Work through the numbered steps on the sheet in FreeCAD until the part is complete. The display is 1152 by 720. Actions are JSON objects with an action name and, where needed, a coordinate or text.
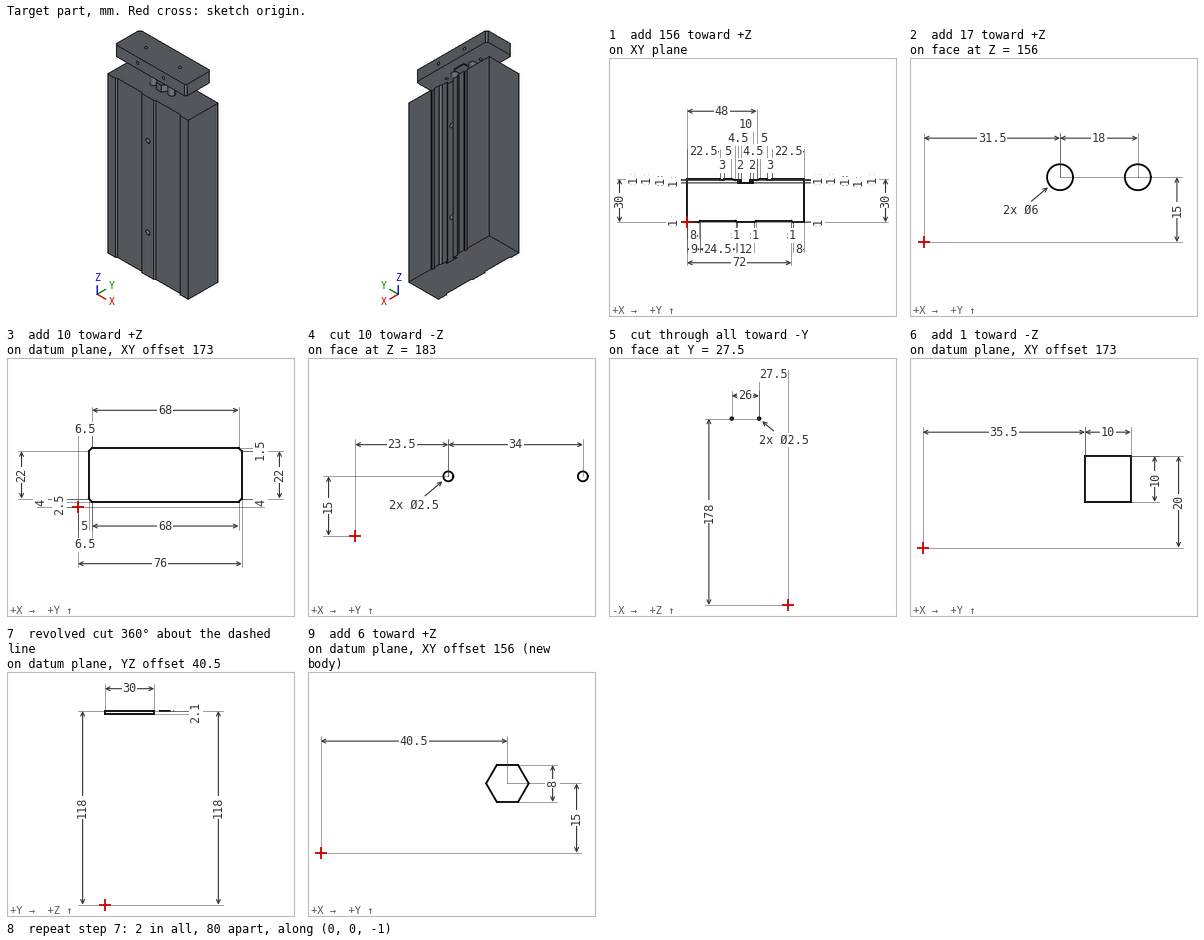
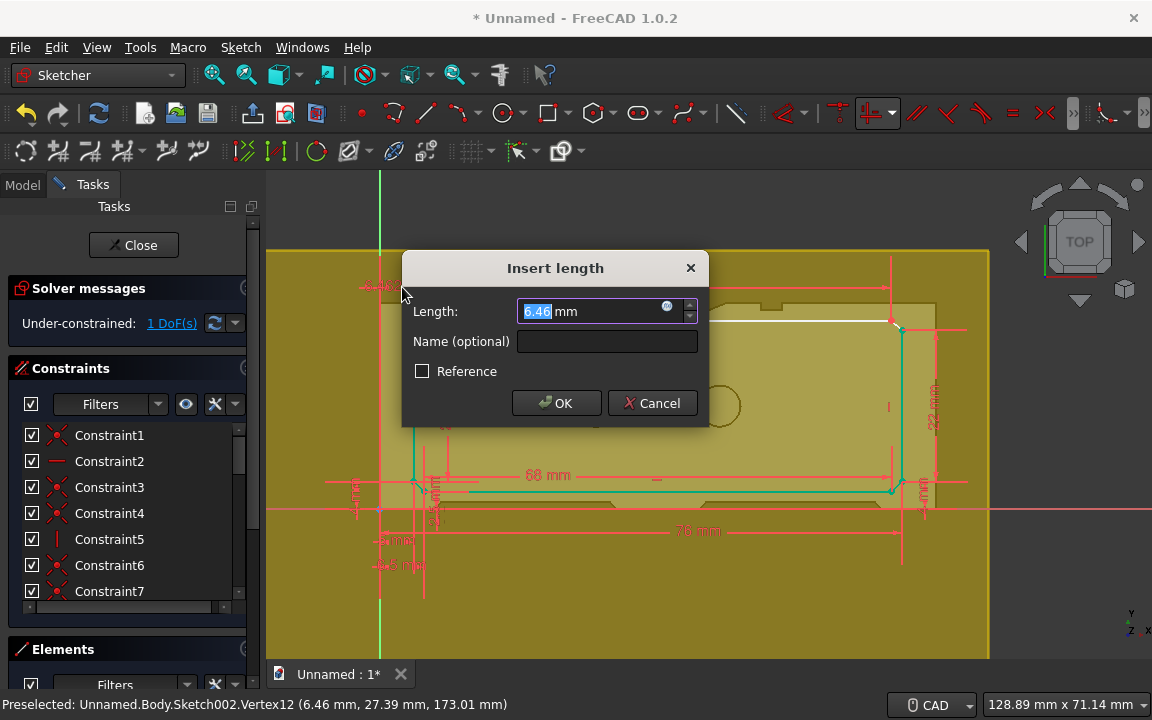
{"action": "type", "text": "6.5"}
{"action": "key", "text": "Return"}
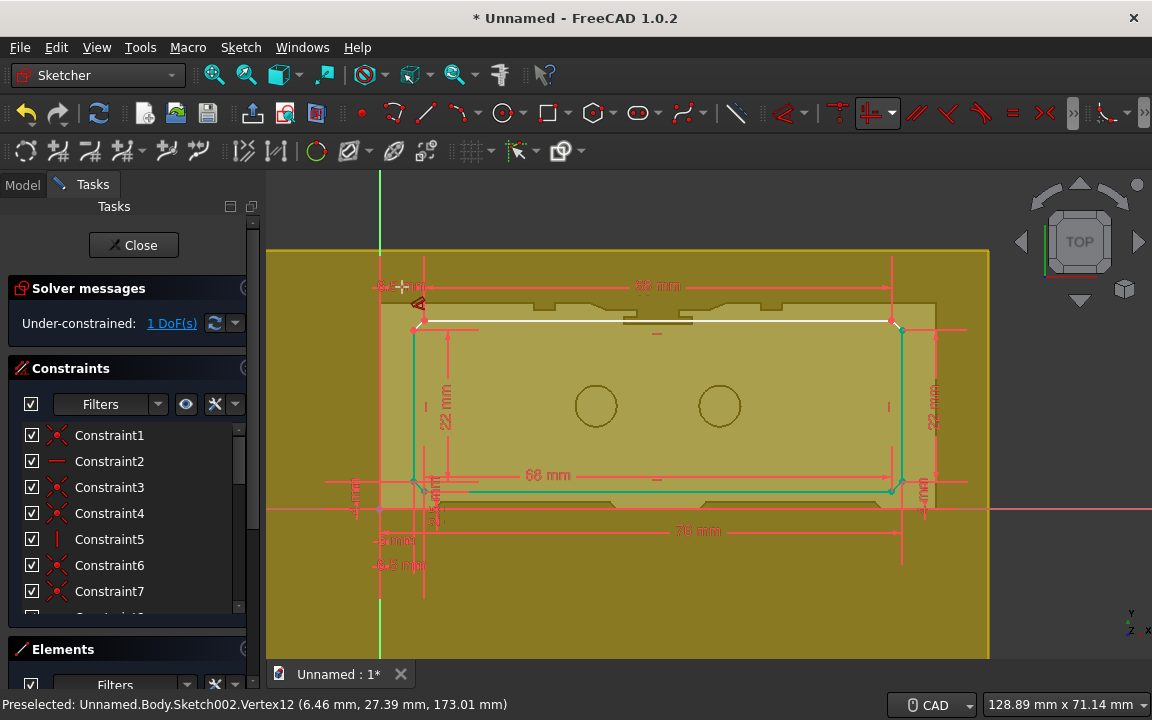
{"action": "scroll", "coordinate": [897, 326], "scroll_direction": "up", "scroll_amount": 7}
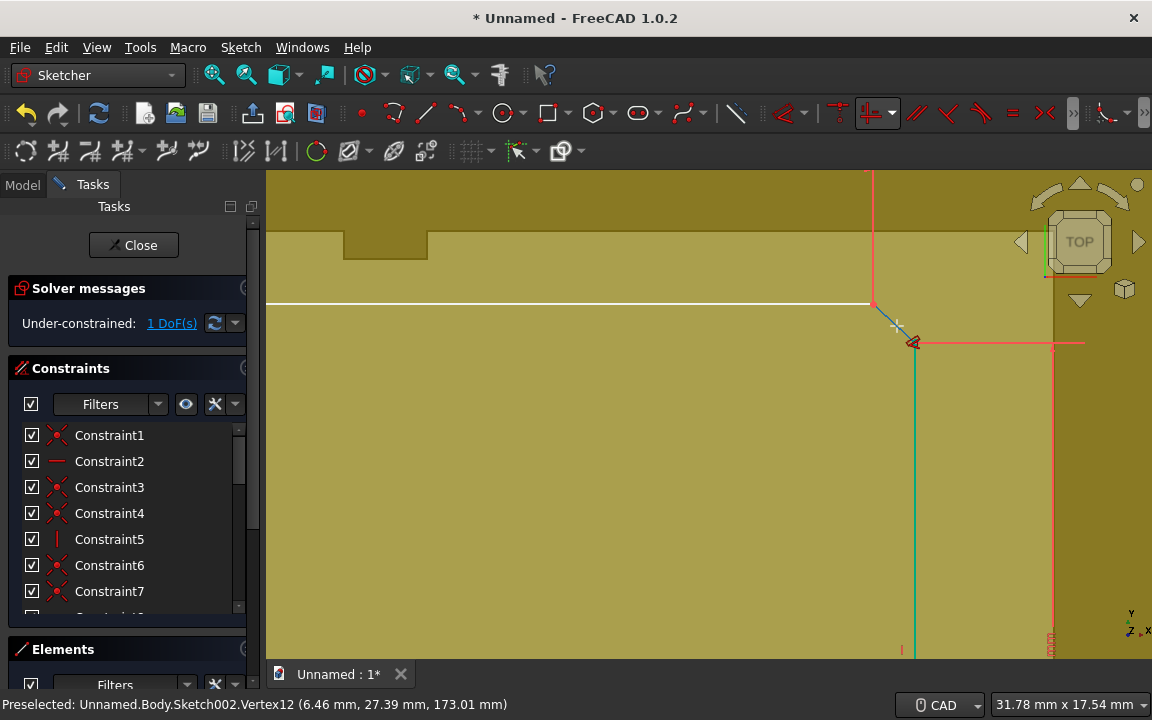
{"action": "left_click", "coordinate": [894, 324]}
{"action": "left_click", "coordinate": [949, 324]}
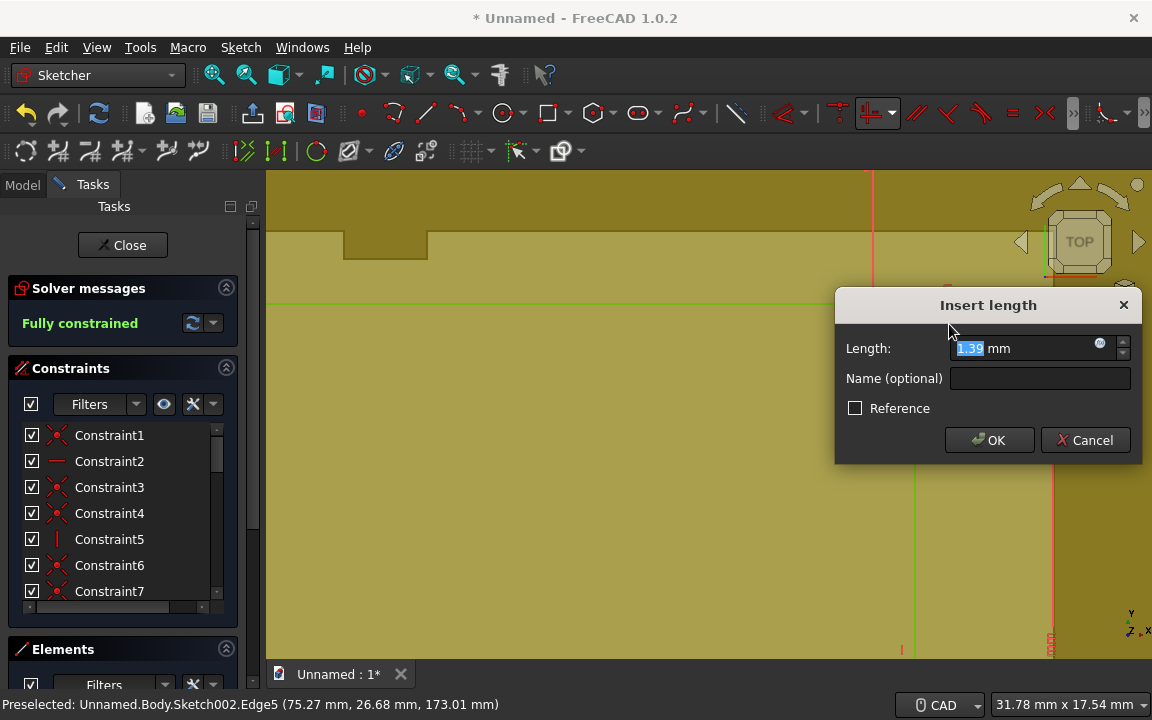
{"action": "type", "text": "1.5"}
{"action": "key", "text": "Return"}
{"action": "key", "text": "Escape"}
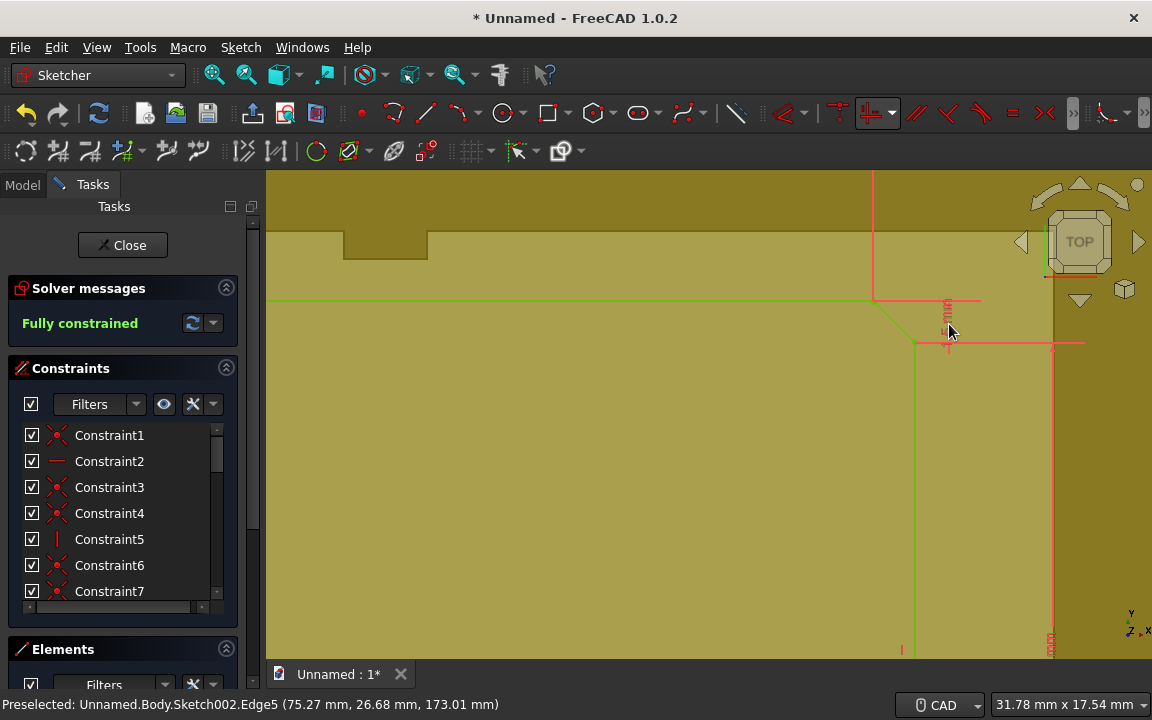
{"action": "left_click", "coordinate": [123, 245]}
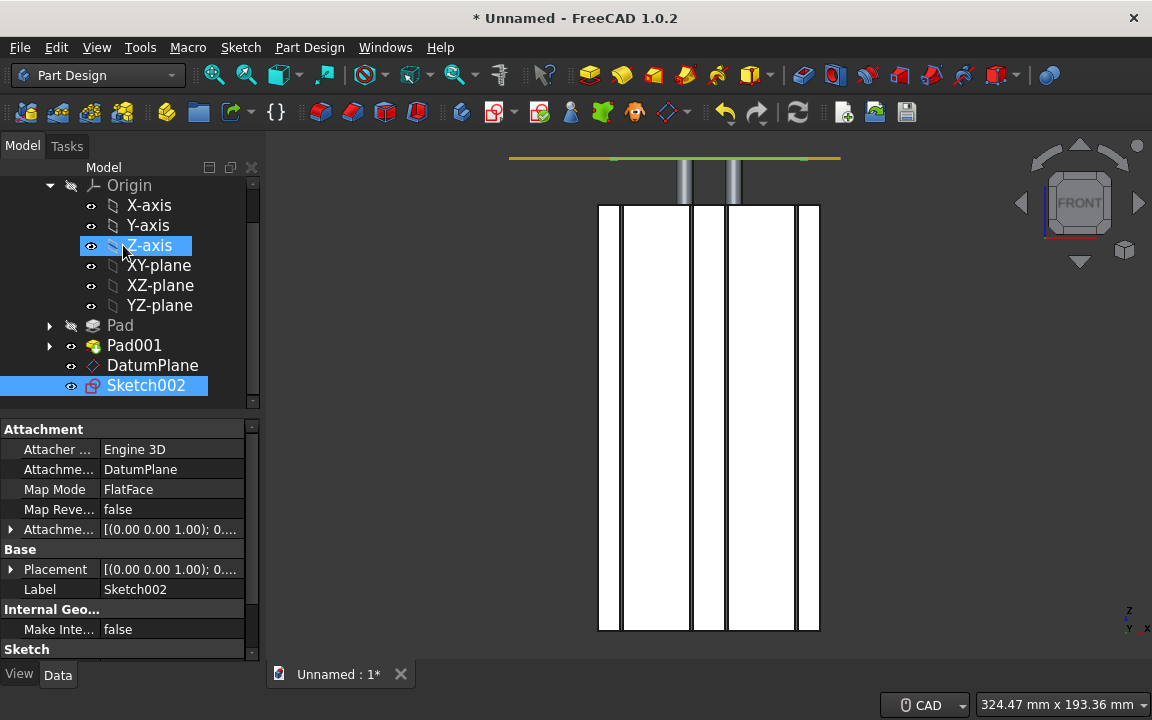
{"action": "left_click", "coordinate": [590, 76]}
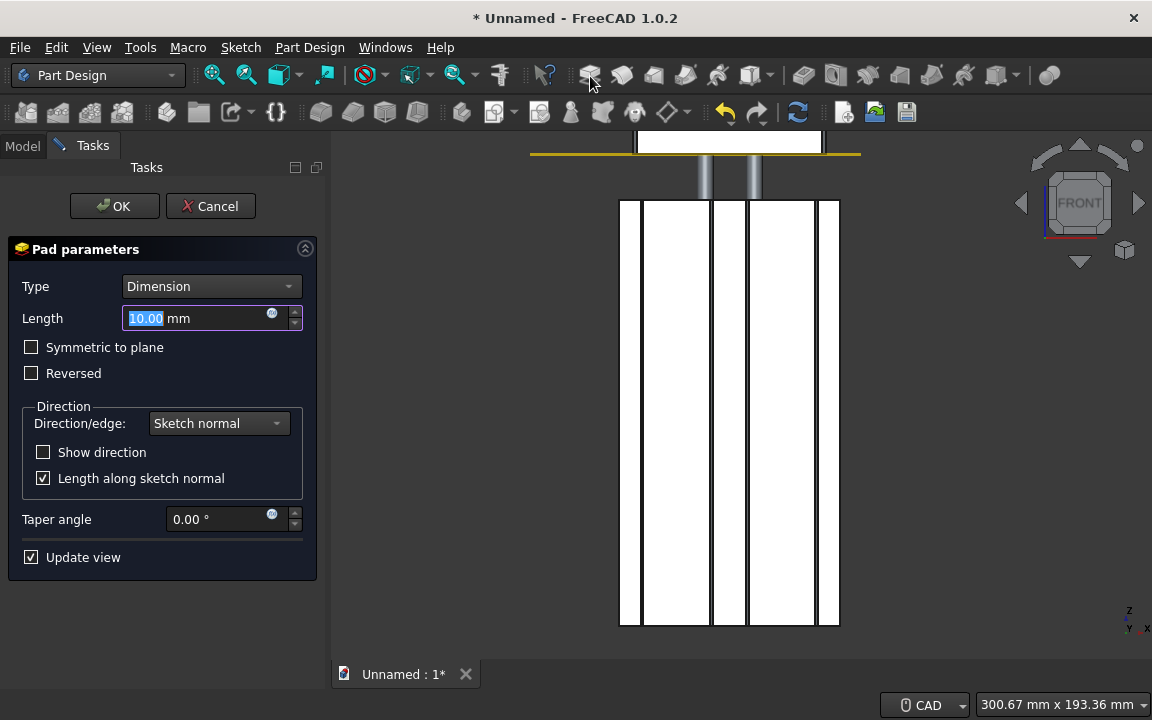
{"action": "type", "text": "10"}
{"action": "key", "text": "Tab"}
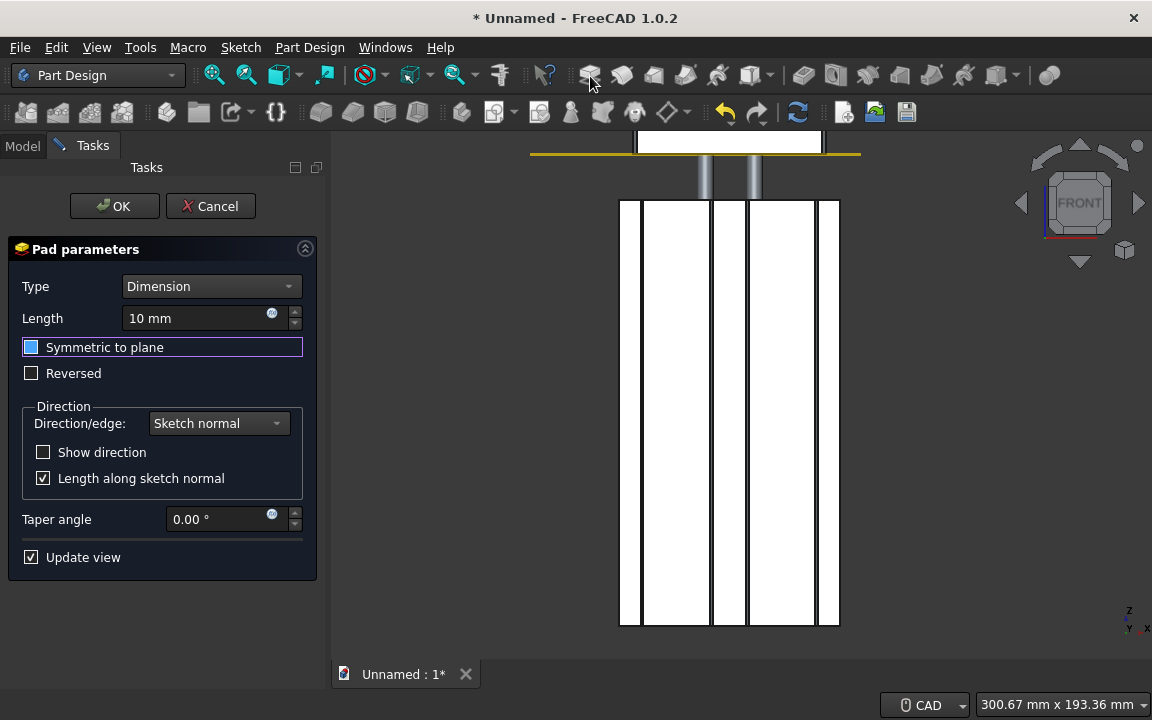
{"action": "left_click", "coordinate": [115, 206]}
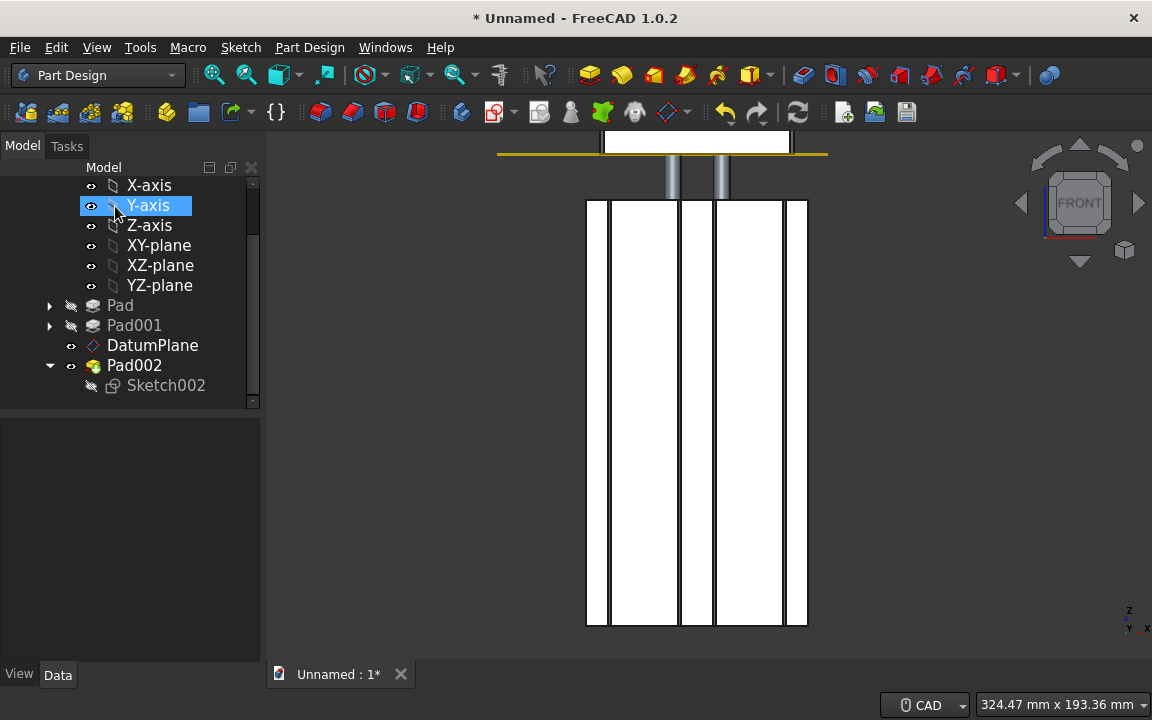
{"action": "left_click", "coordinate": [116, 346]}
{"action": "key", "text": "space"}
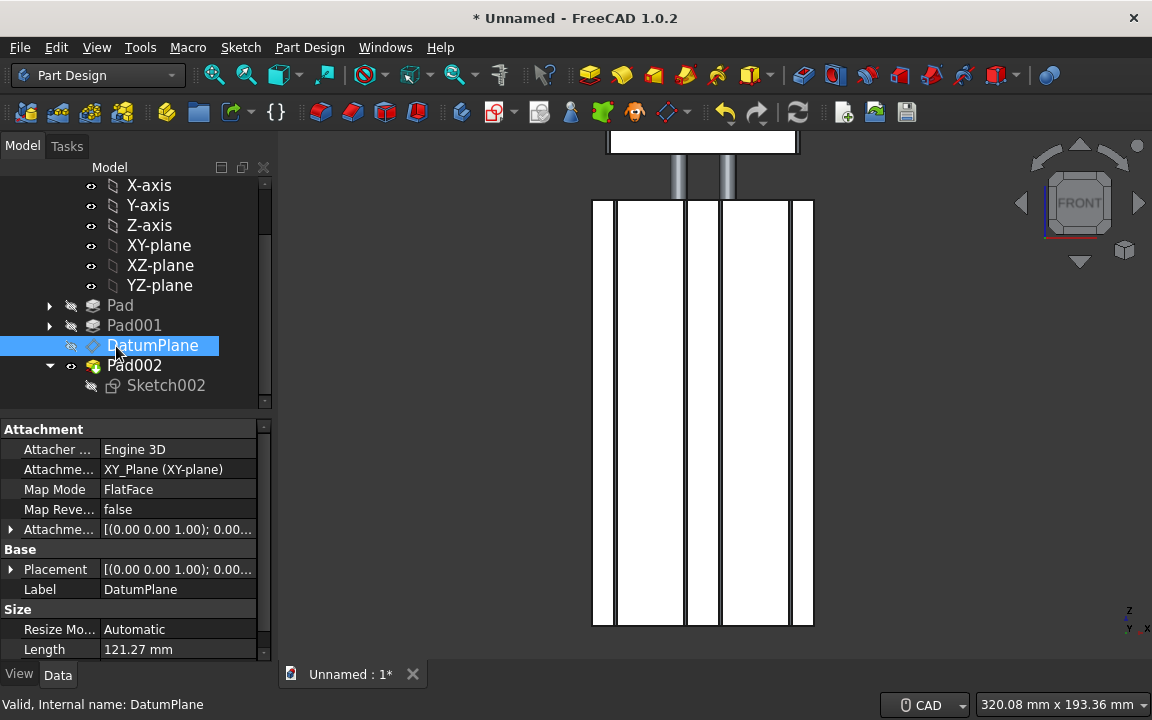
{"action": "key", "text": "v f"}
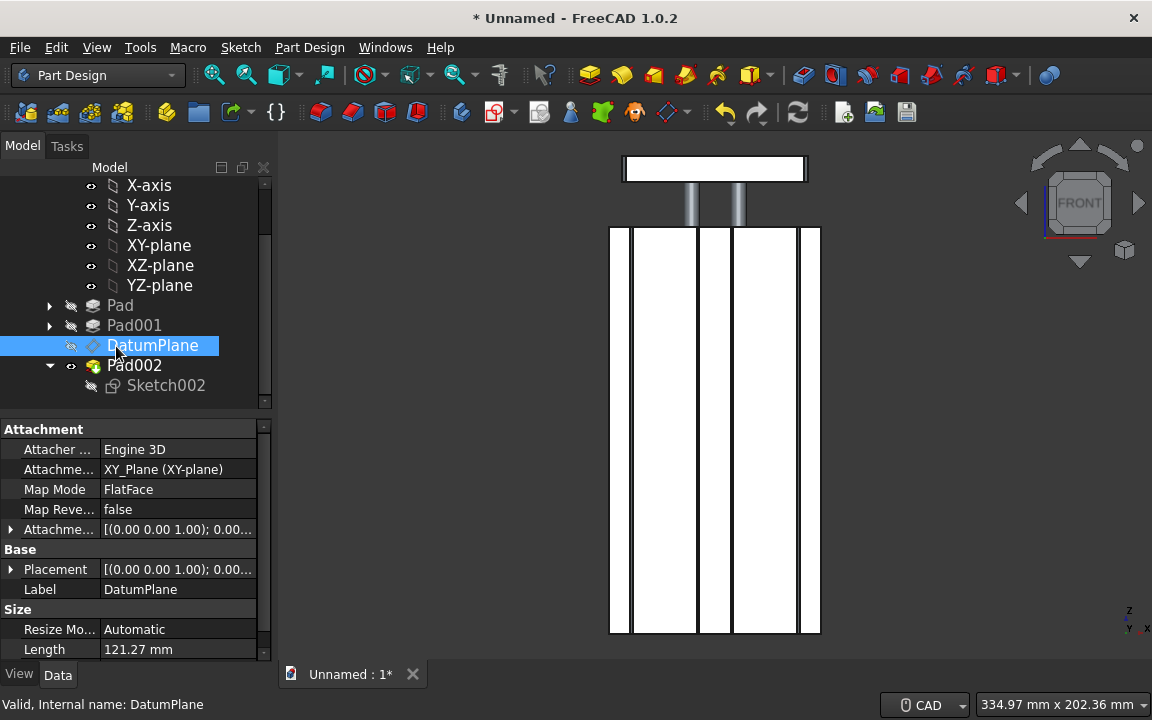
{"action": "key", "text": "0"}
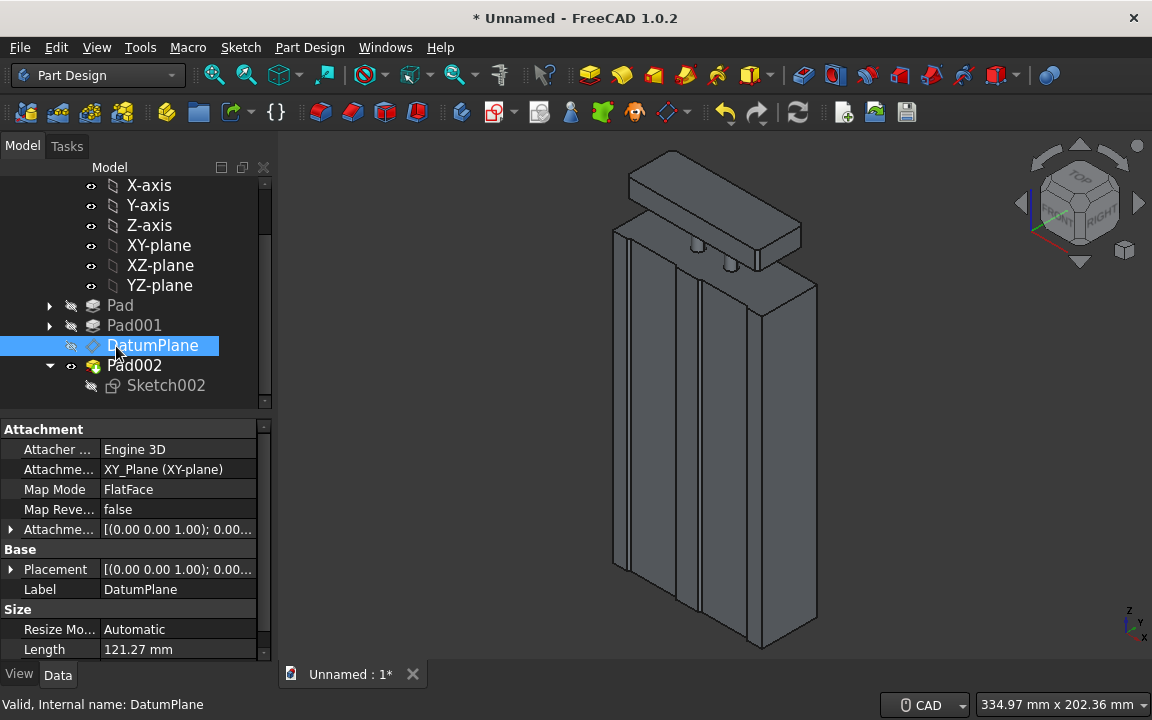
{"action": "left_click", "coordinate": [752, 221]}